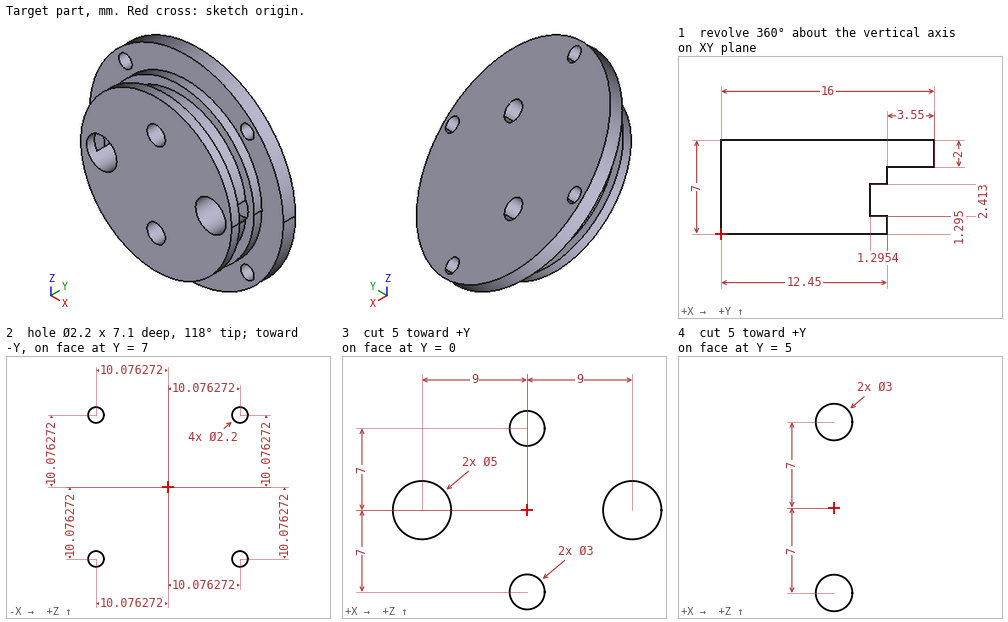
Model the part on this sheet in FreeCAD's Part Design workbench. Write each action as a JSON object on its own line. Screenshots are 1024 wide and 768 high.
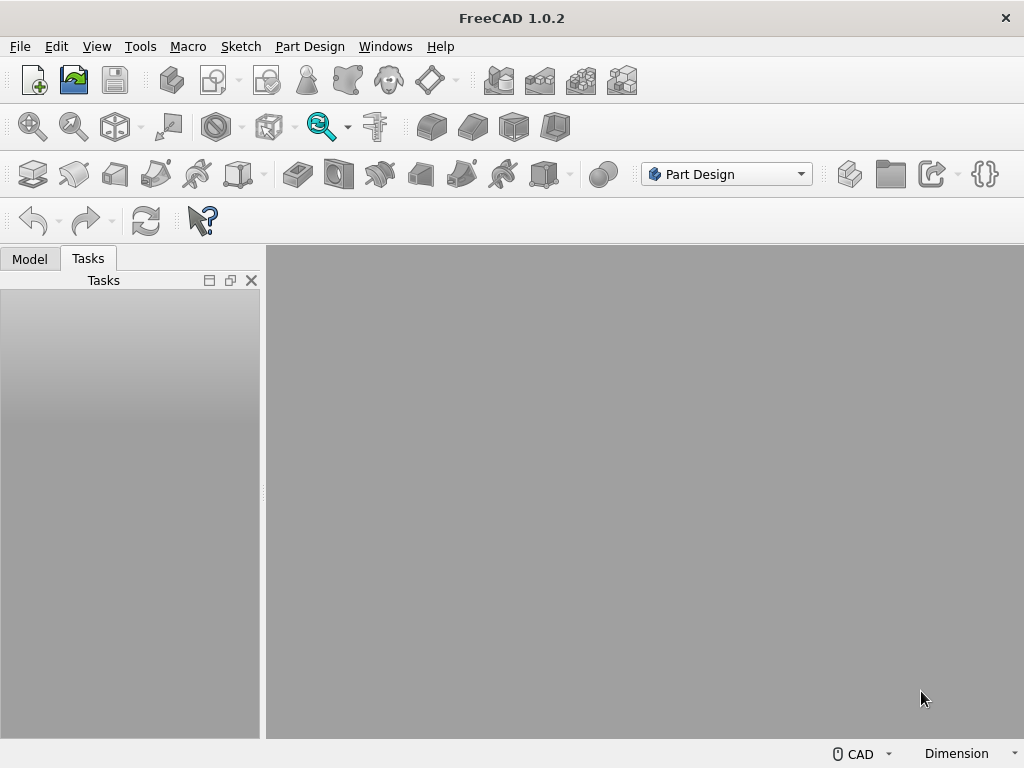
{"action": "left_click", "coordinate": [33, 80]}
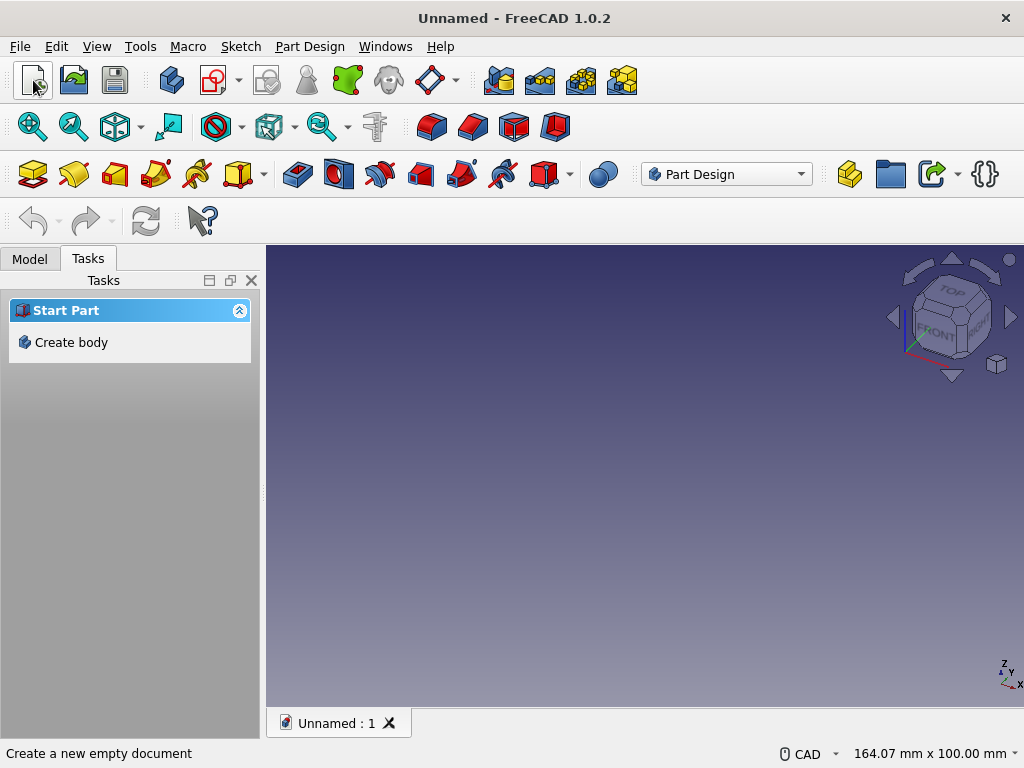
{"action": "left_click", "coordinate": [212, 80]}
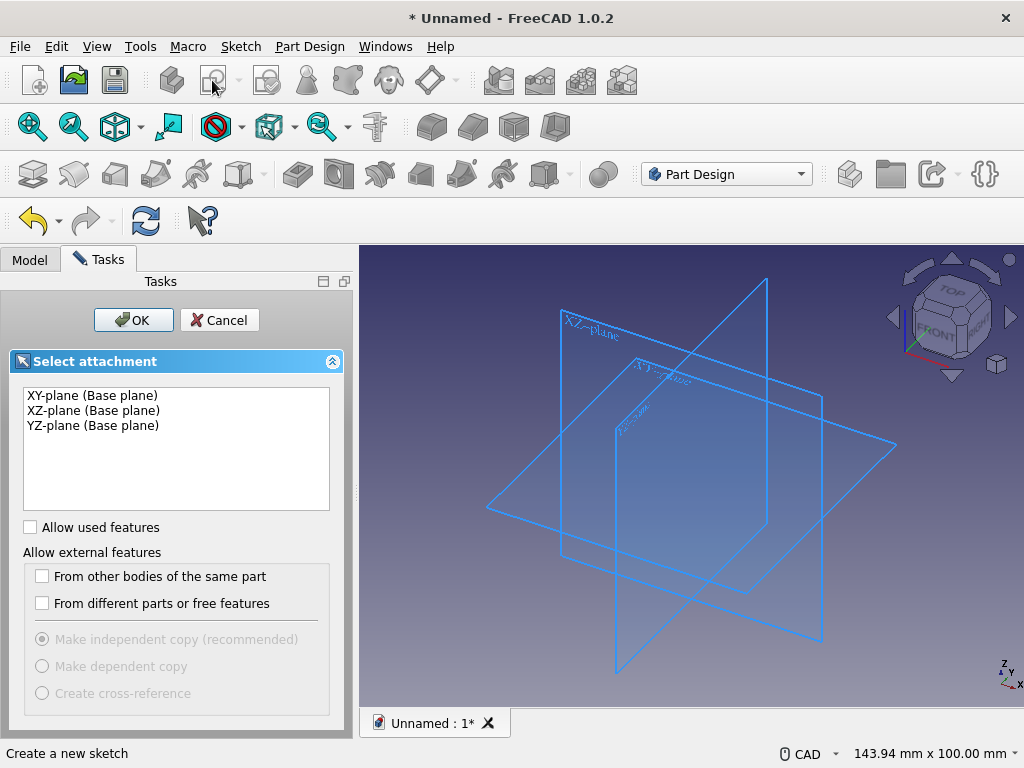
{"action": "left_click", "coordinate": [84, 396]}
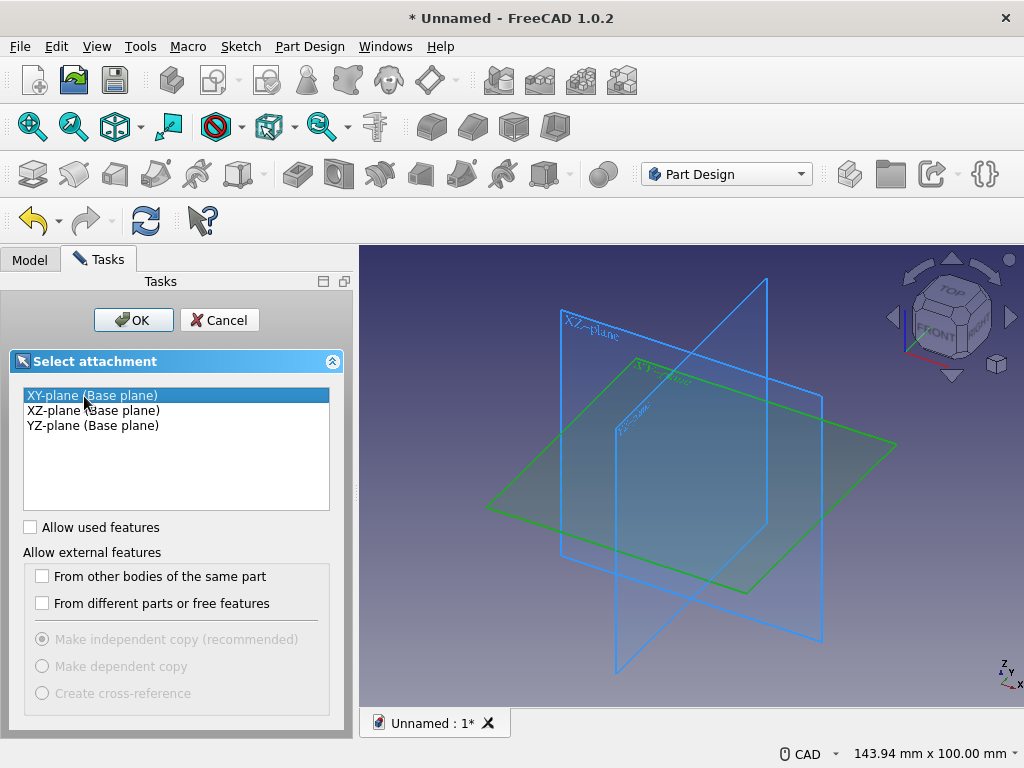
{"action": "left_click", "coordinate": [134, 320]}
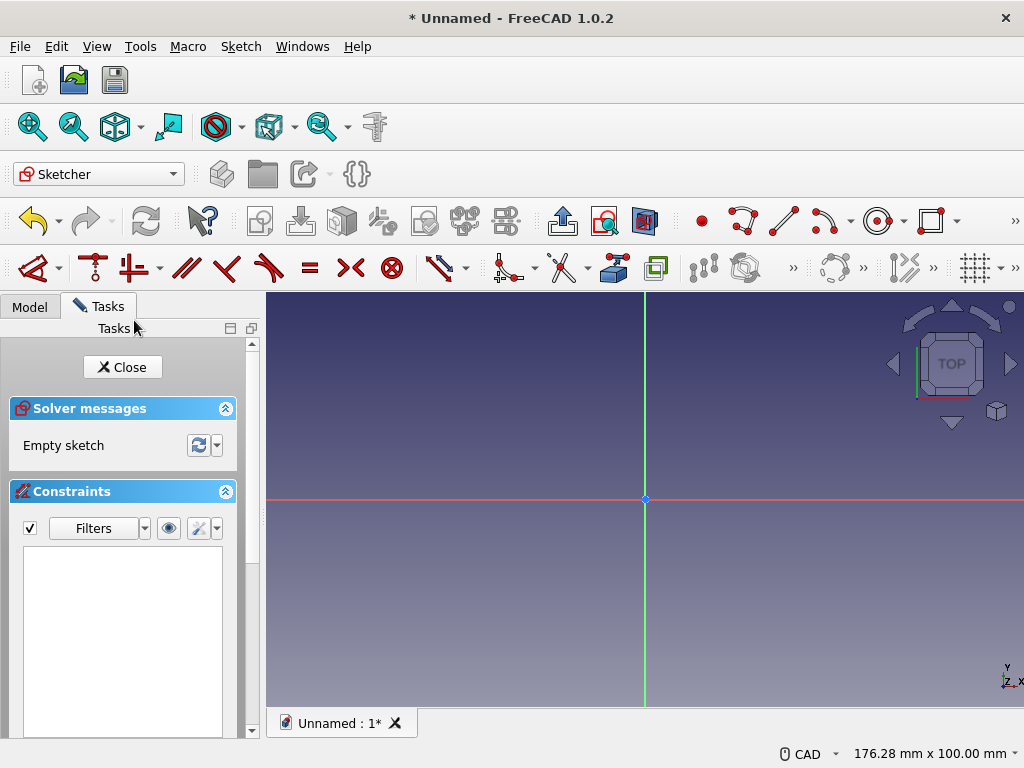
{"action": "scroll", "coordinate": [698, 482], "scroll_direction": "up", "scroll_amount": 9}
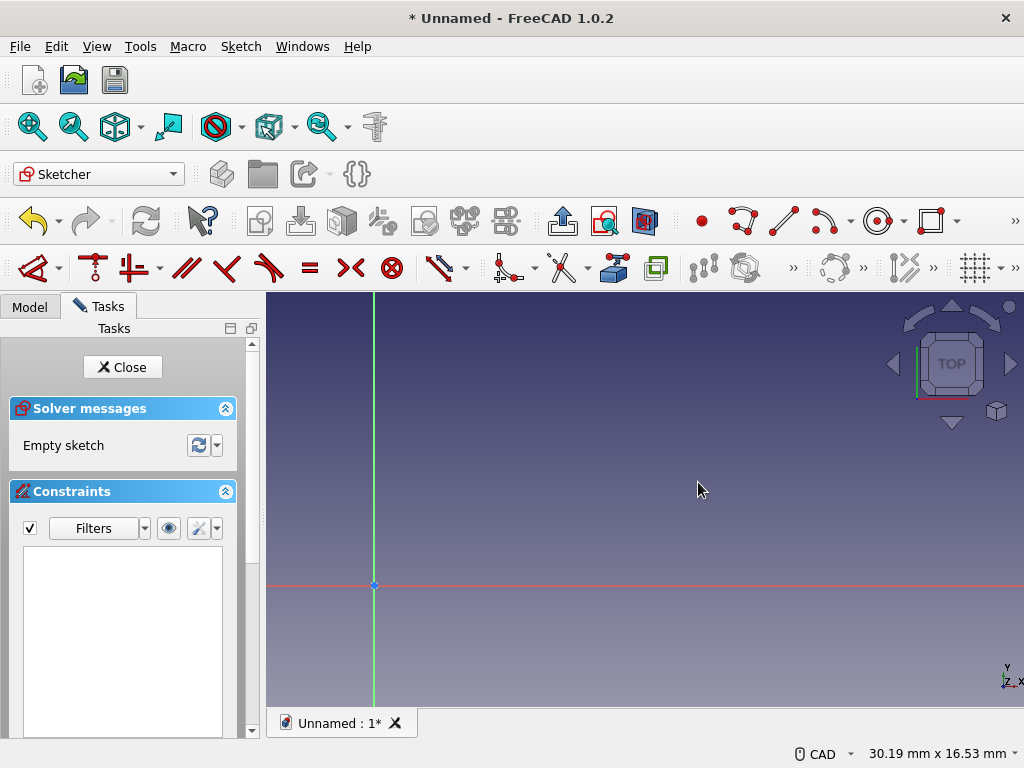
{"action": "left_click", "coordinate": [743, 222]}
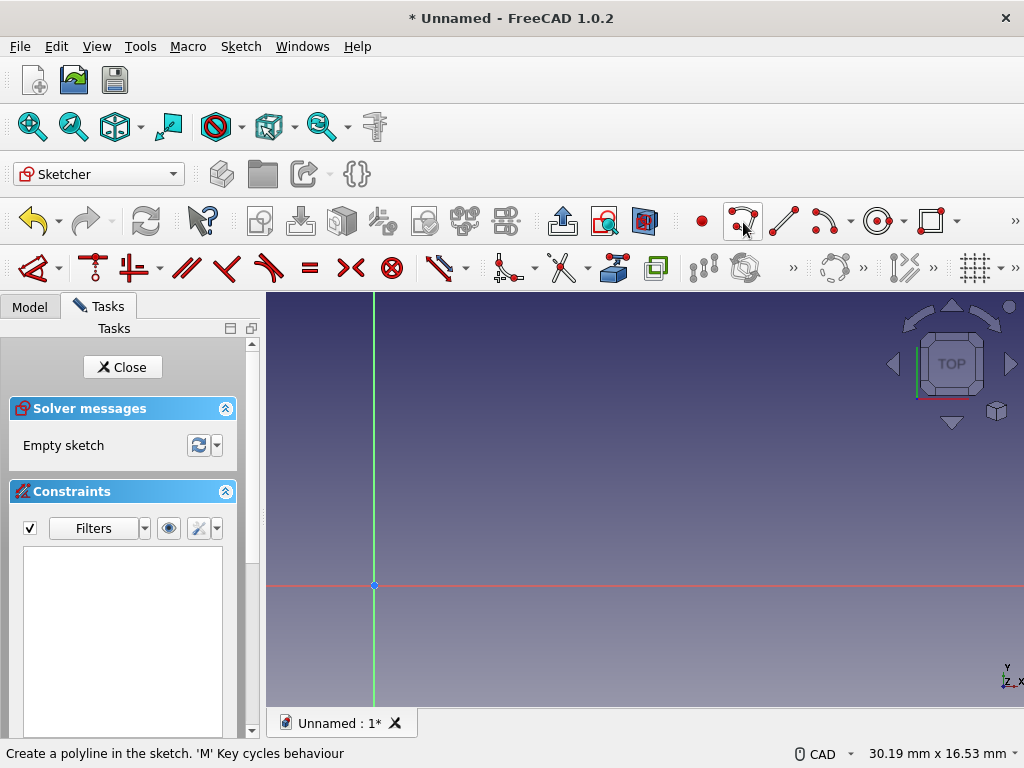
{"action": "left_click", "coordinate": [374, 586]}
{"action": "left_click", "coordinate": [687, 577]}
{"action": "left_click", "coordinate": [687, 553]}
{"action": "left_click", "coordinate": [655, 553]}
{"action": "left_click", "coordinate": [655, 492]}
{"action": "left_click", "coordinate": [687, 492]}
{"action": "left_click", "coordinate": [687, 460]}
{"action": "left_click", "coordinate": [776, 460]}
{"action": "left_click", "coordinate": [776, 410]}
{"action": "left_click", "coordinate": [383, 410]}
{"action": "left_click", "coordinate": [374, 586]}
{"action": "key", "text": "Escape"}
{"action": "key", "text": "Escape"}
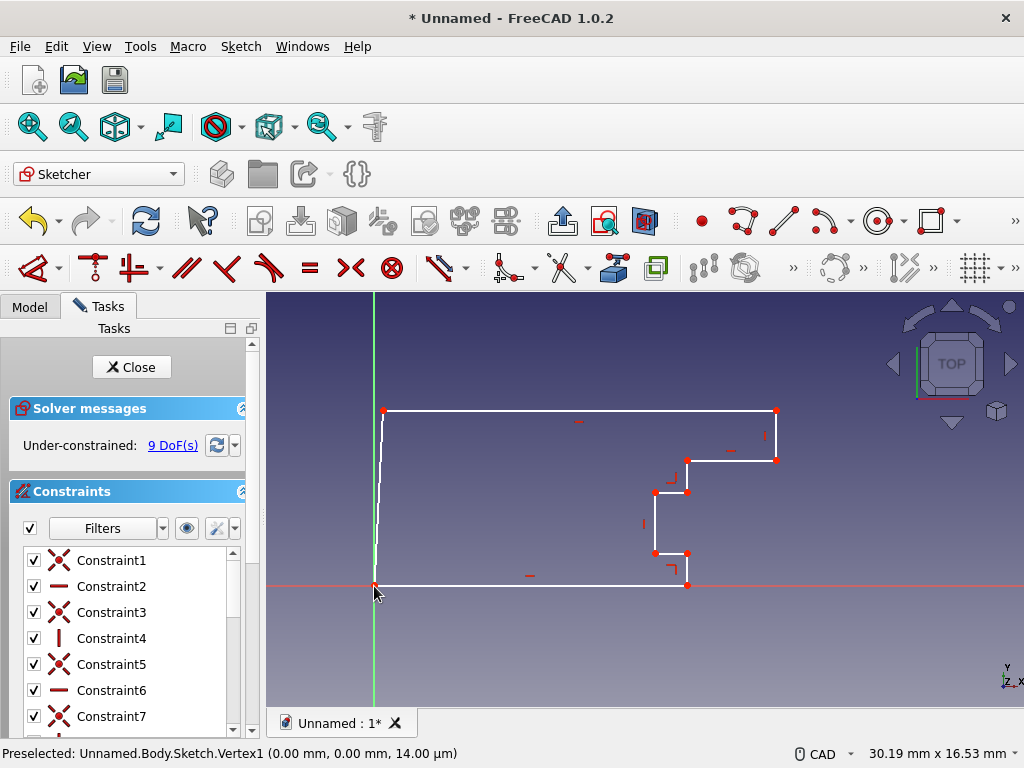
{"action": "left_click", "coordinate": [377, 533]}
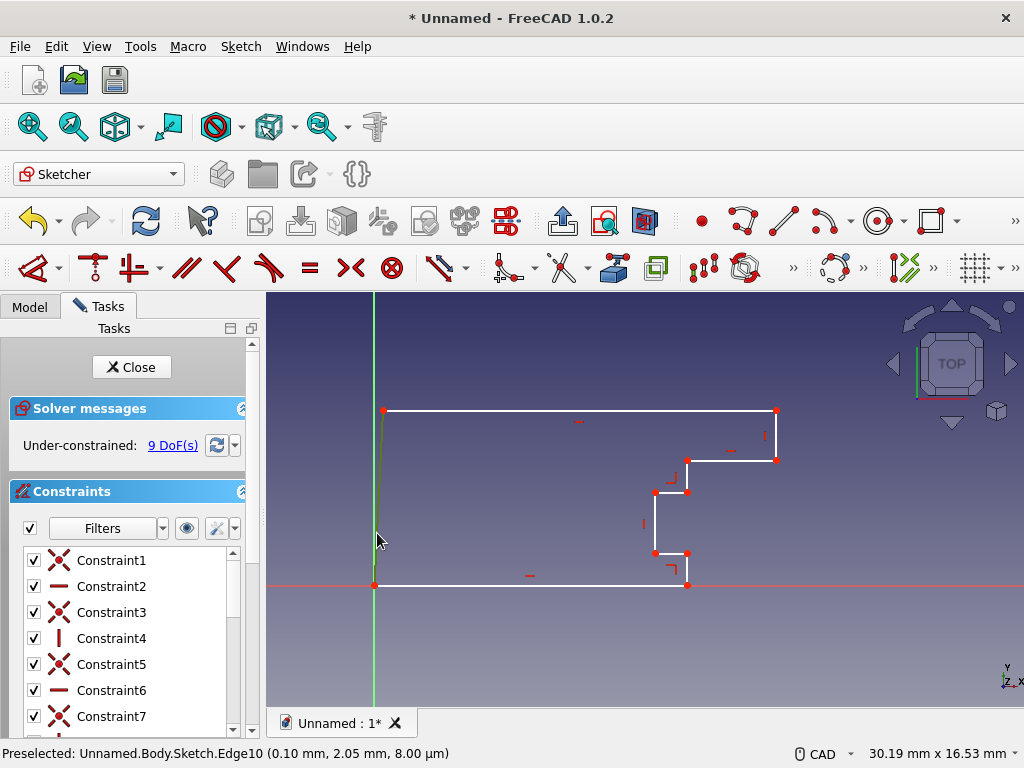
{"action": "left_click", "coordinate": [160, 268]}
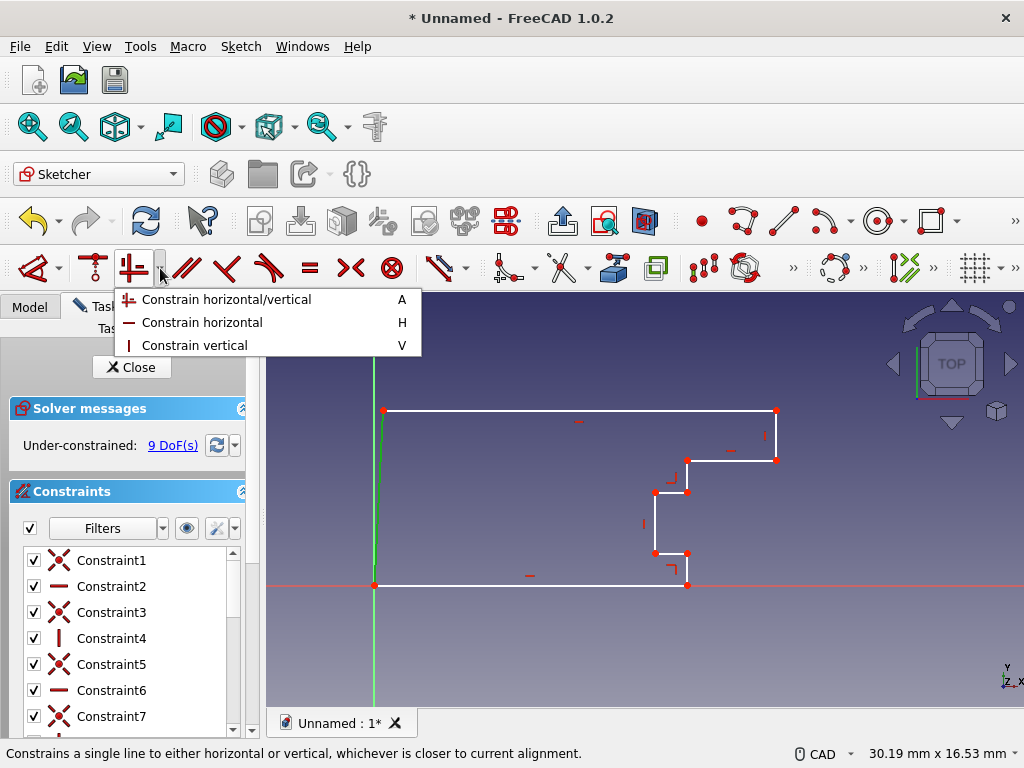
{"action": "left_click", "coordinate": [268, 346]}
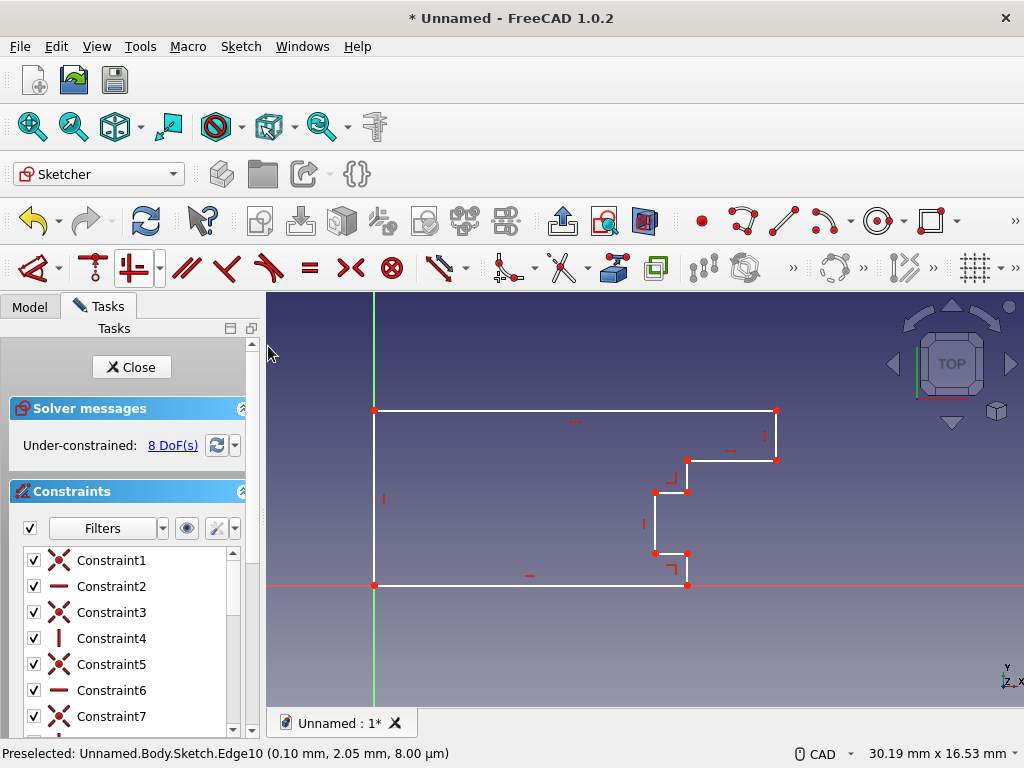
{"action": "left_click", "coordinate": [776, 446]}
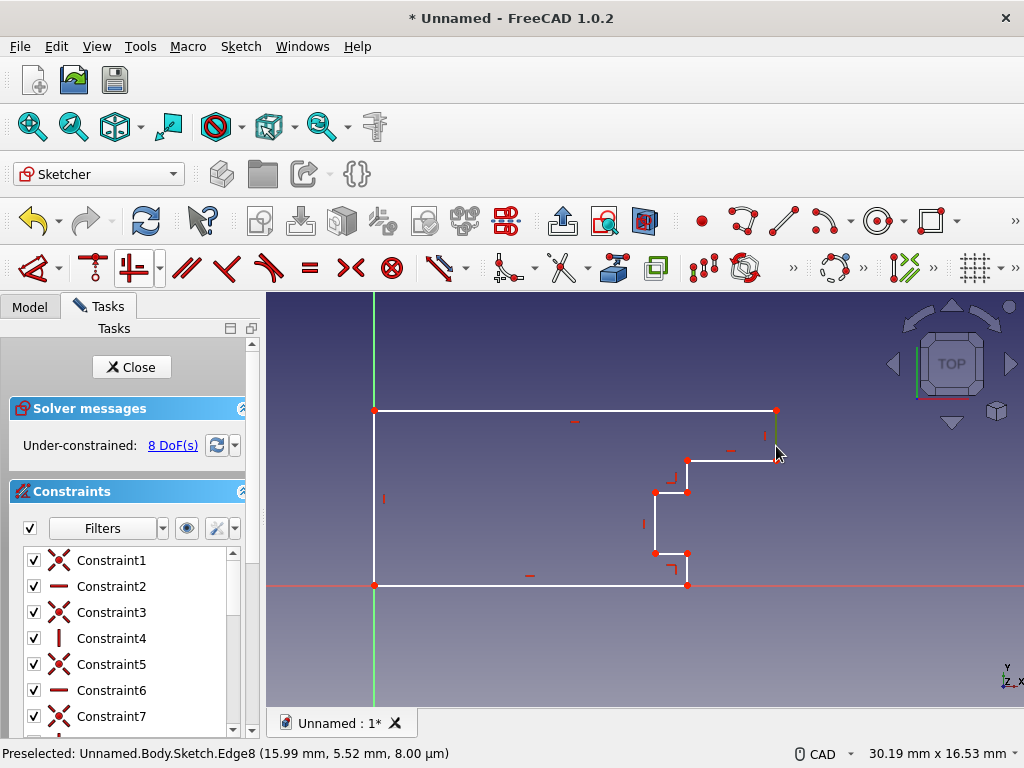
{"action": "key", "text": "i"}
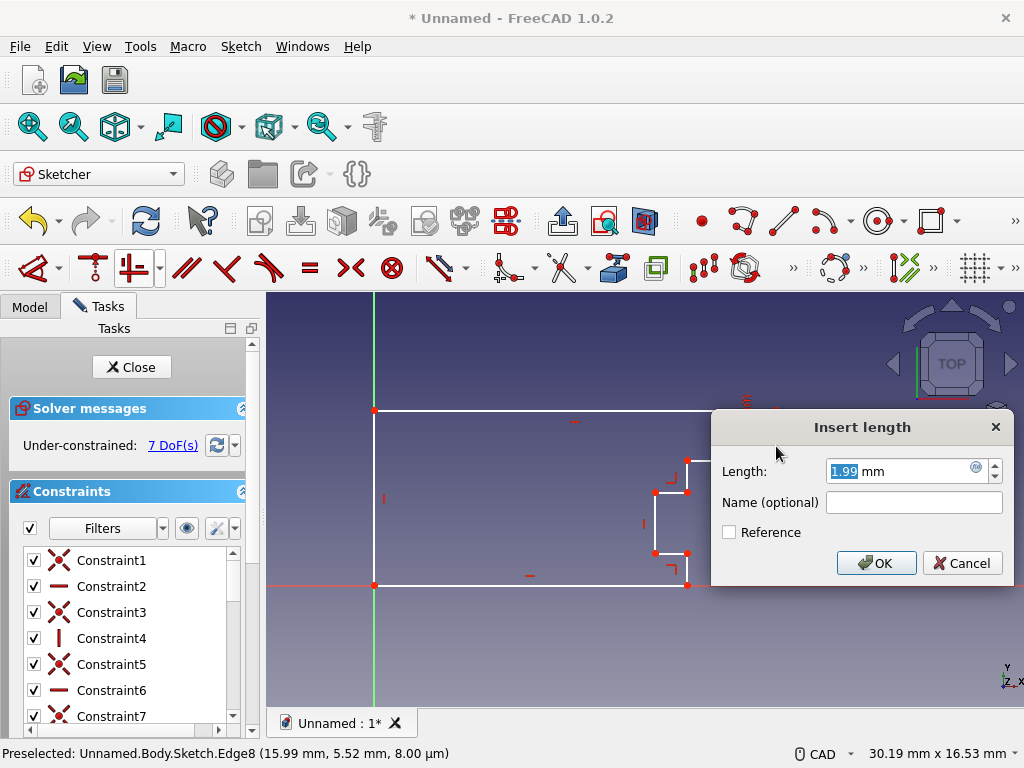
{"action": "type", "text": "2"}
{"action": "key", "text": "Return"}